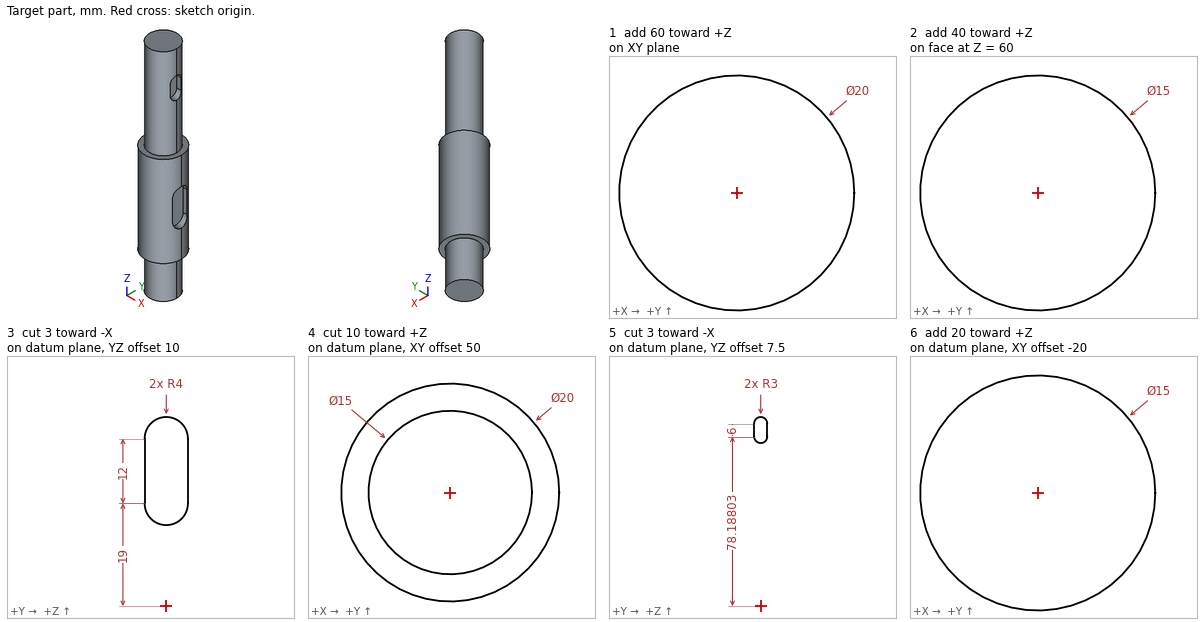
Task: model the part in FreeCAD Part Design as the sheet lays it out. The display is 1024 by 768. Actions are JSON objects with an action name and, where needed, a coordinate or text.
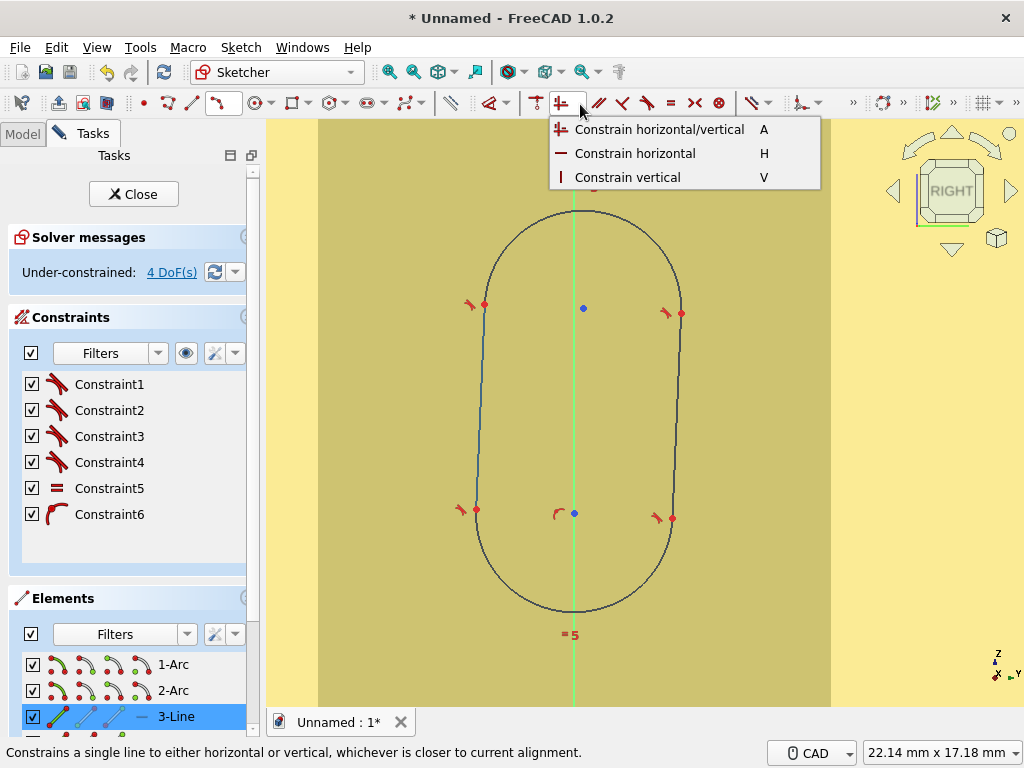
{"action": "left_click", "coordinate": [685, 177]}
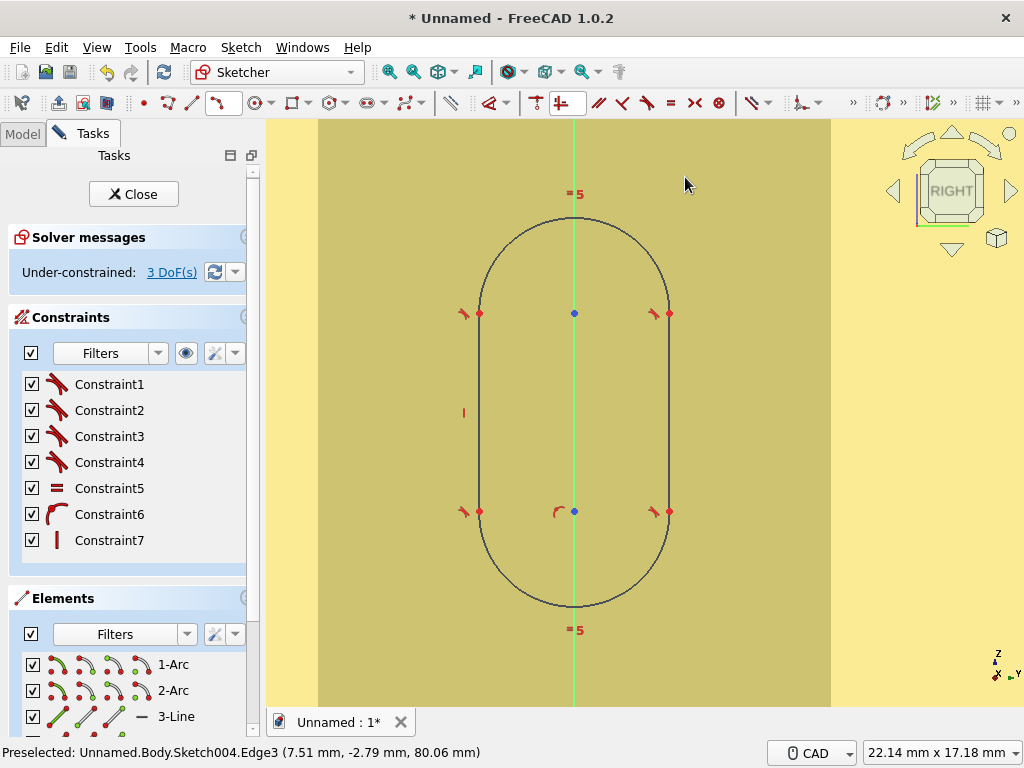
{"action": "left_click", "coordinate": [490, 104]}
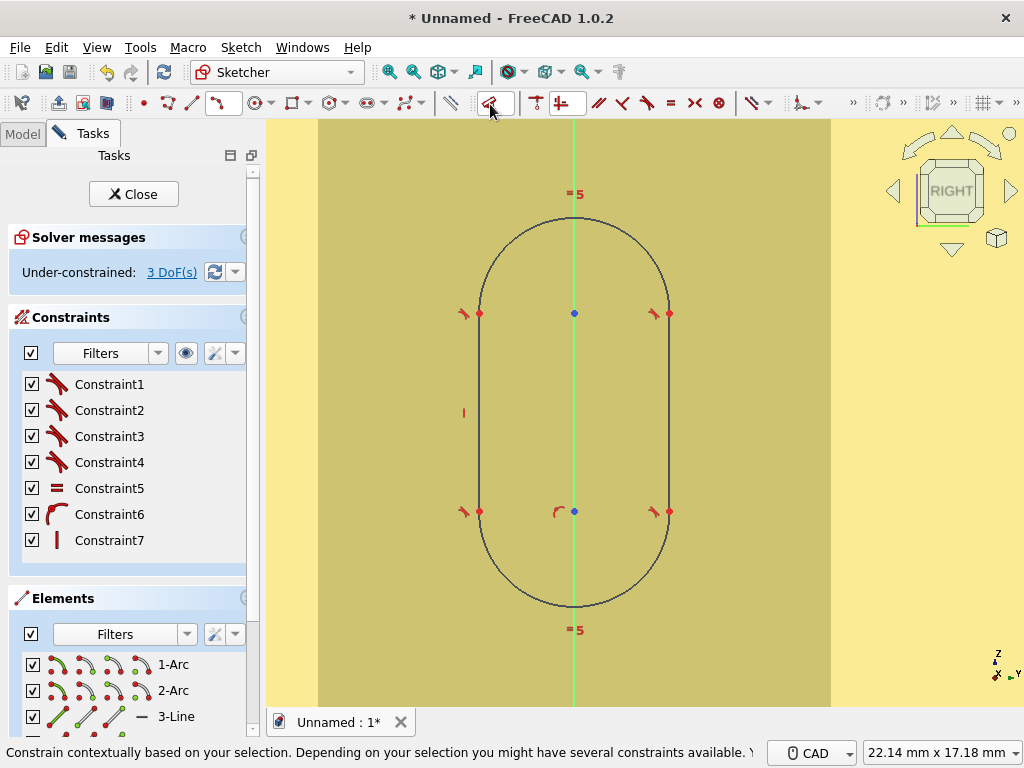
{"action": "left_click", "coordinate": [518, 589]}
{"action": "left_click", "coordinate": [499, 615]}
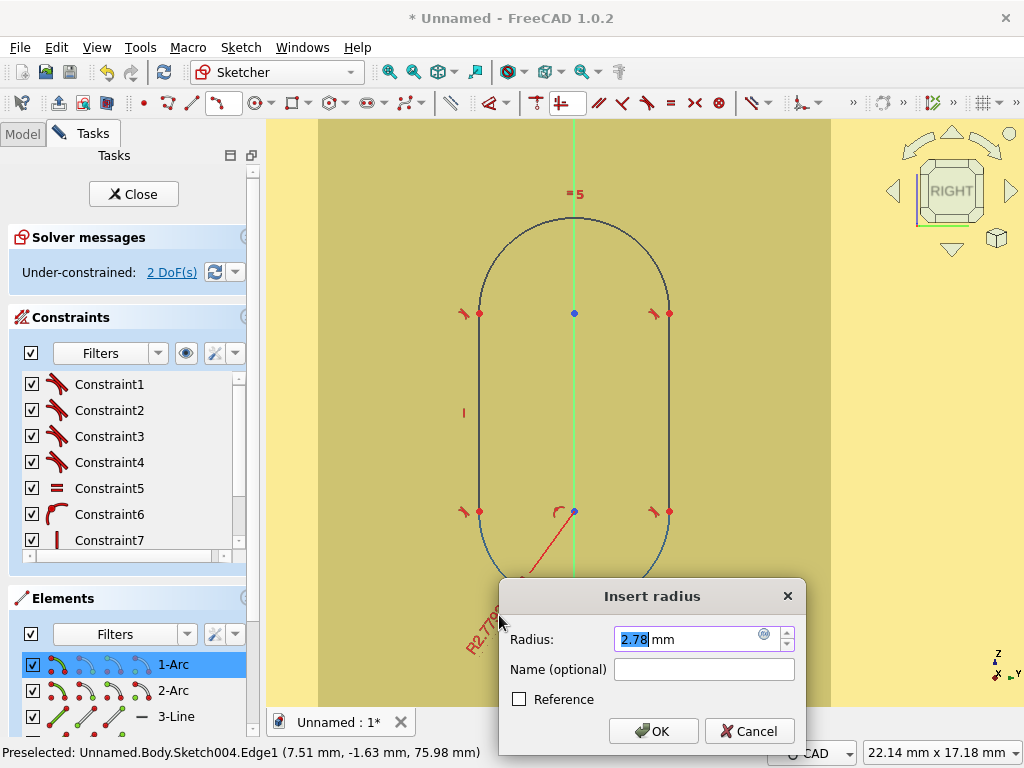
{"action": "type", "text": "3"}
{"action": "key", "text": "Return"}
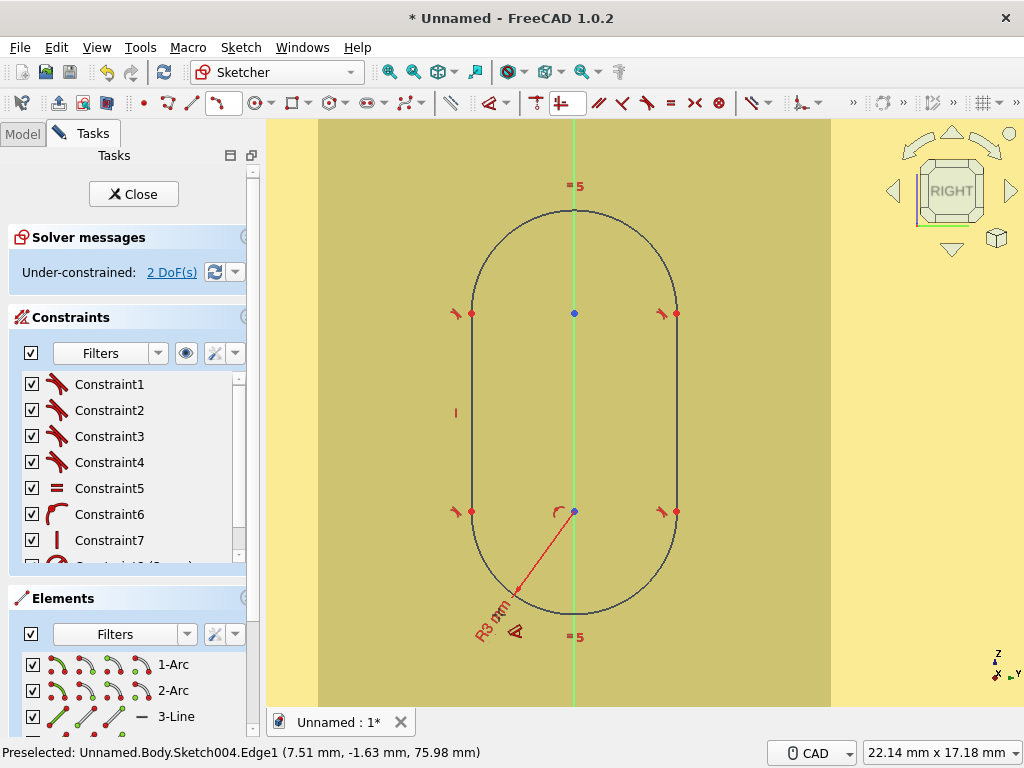
{"action": "left_click", "coordinate": [472, 452]}
{"action": "left_click", "coordinate": [438, 412]}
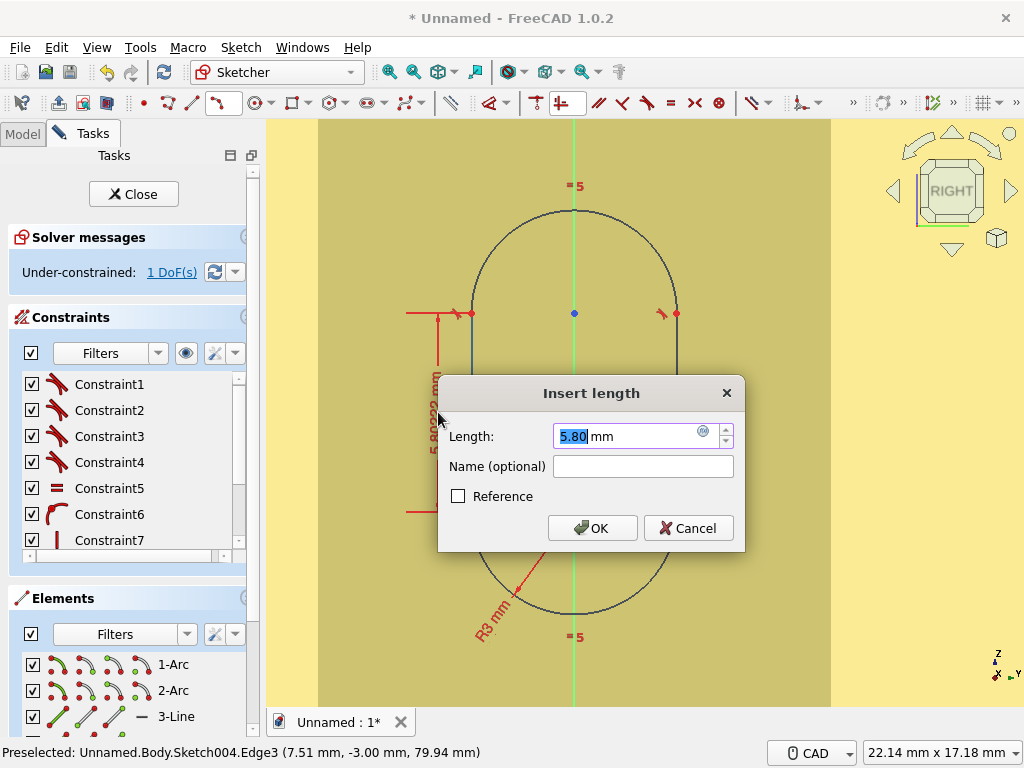
{"action": "type", "text": "6"}
{"action": "key", "text": "Return"}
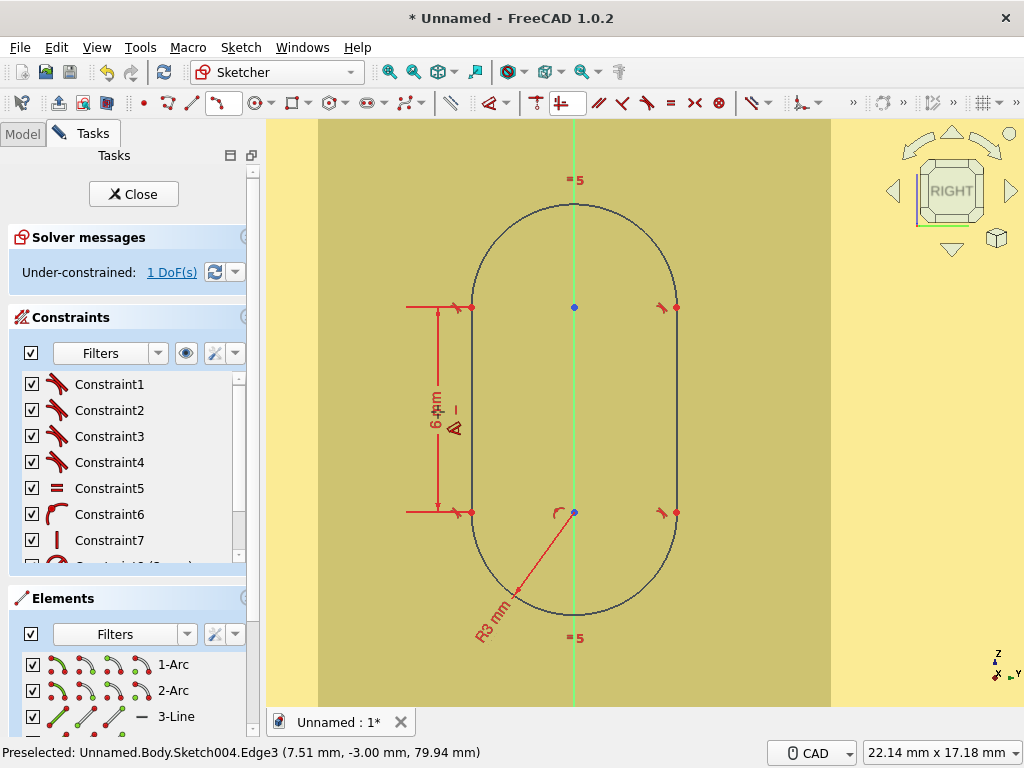
{"action": "left_click", "coordinate": [472, 512]}
{"action": "left_click", "coordinate": [438, 557]}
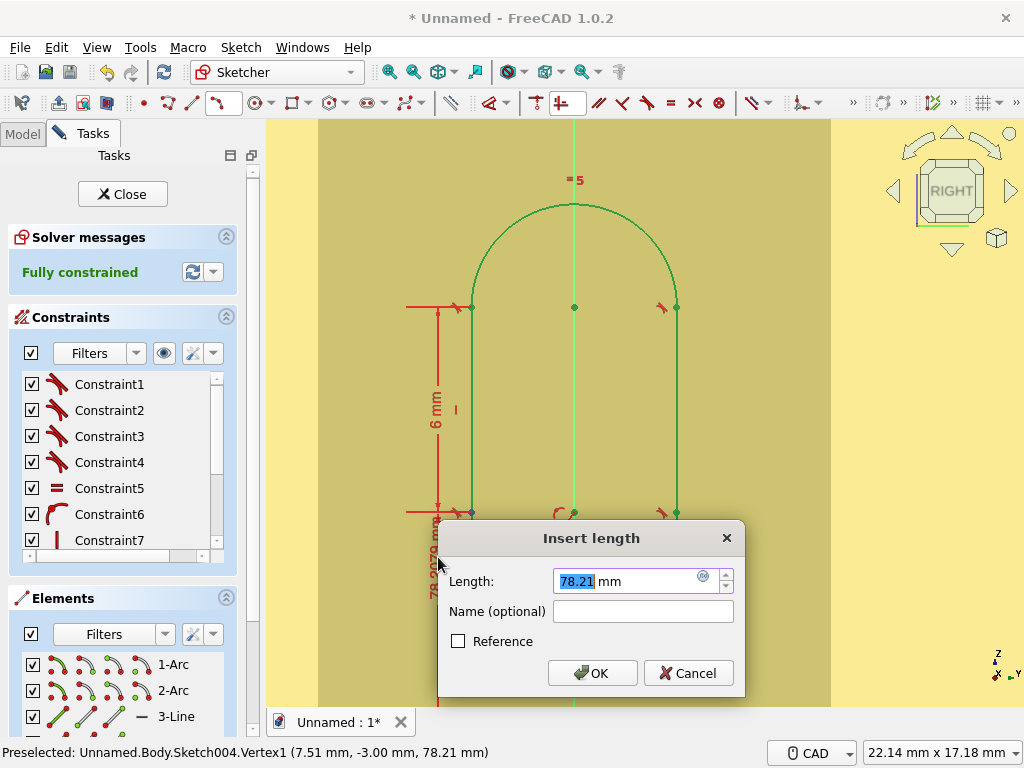
{"action": "type", "text": "78.18803"}
{"action": "key", "text": "Return"}
{"action": "key", "text": "Escape"}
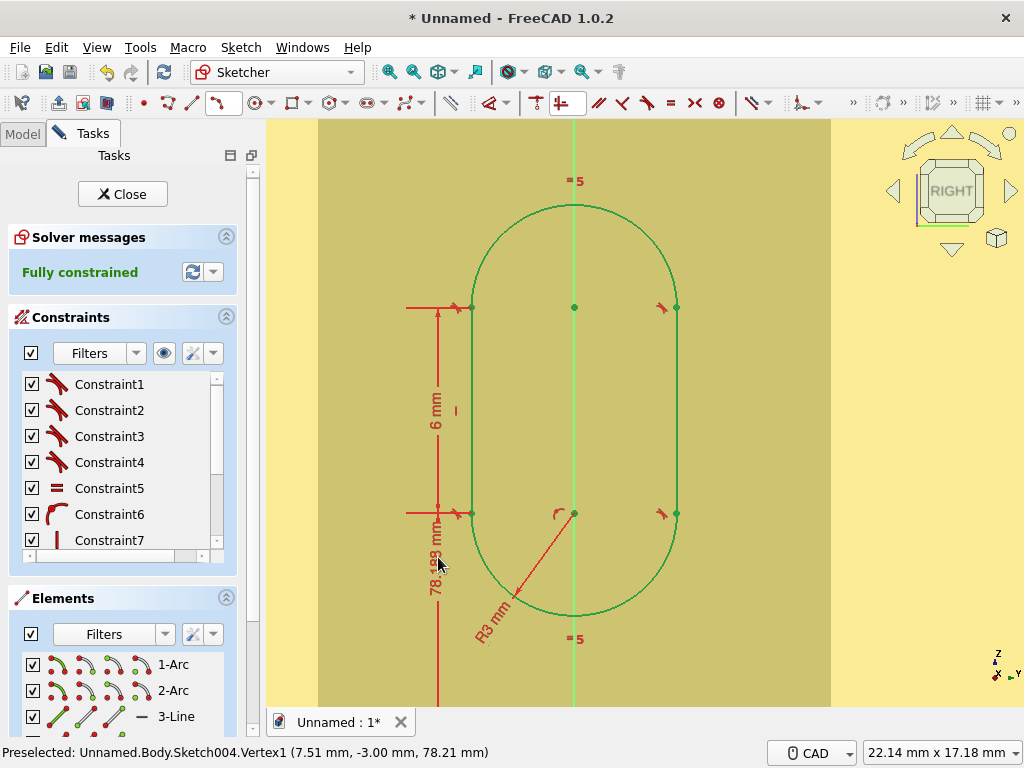
{"action": "left_click", "coordinate": [123, 194]}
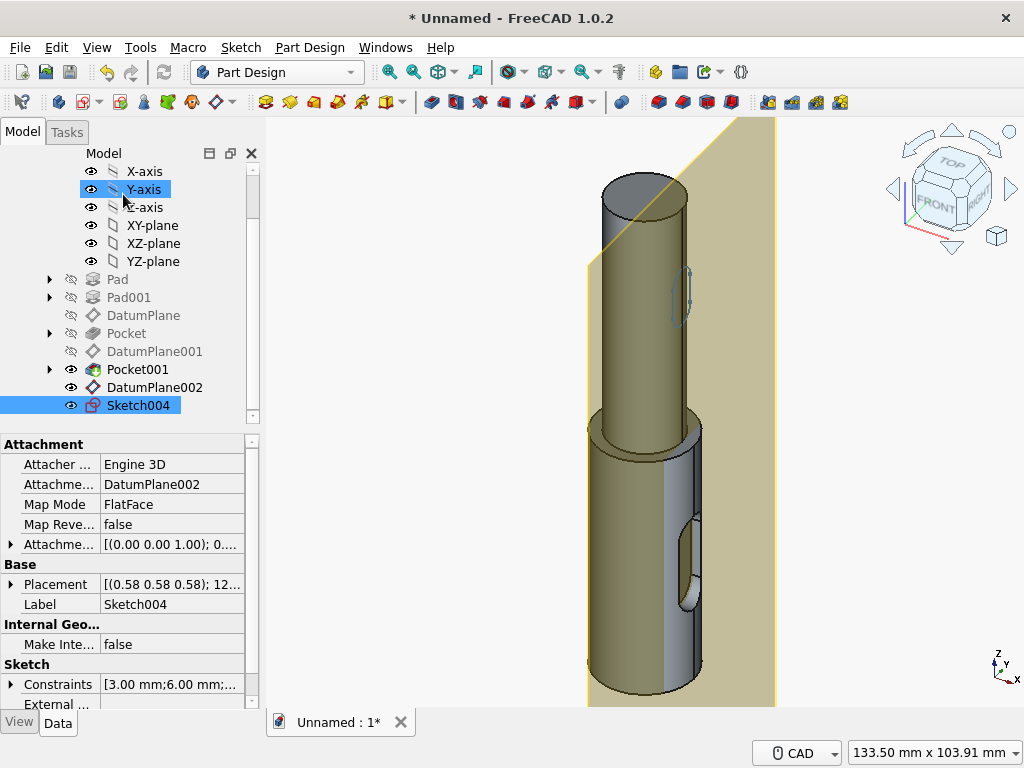
{"action": "left_click", "coordinate": [432, 102]}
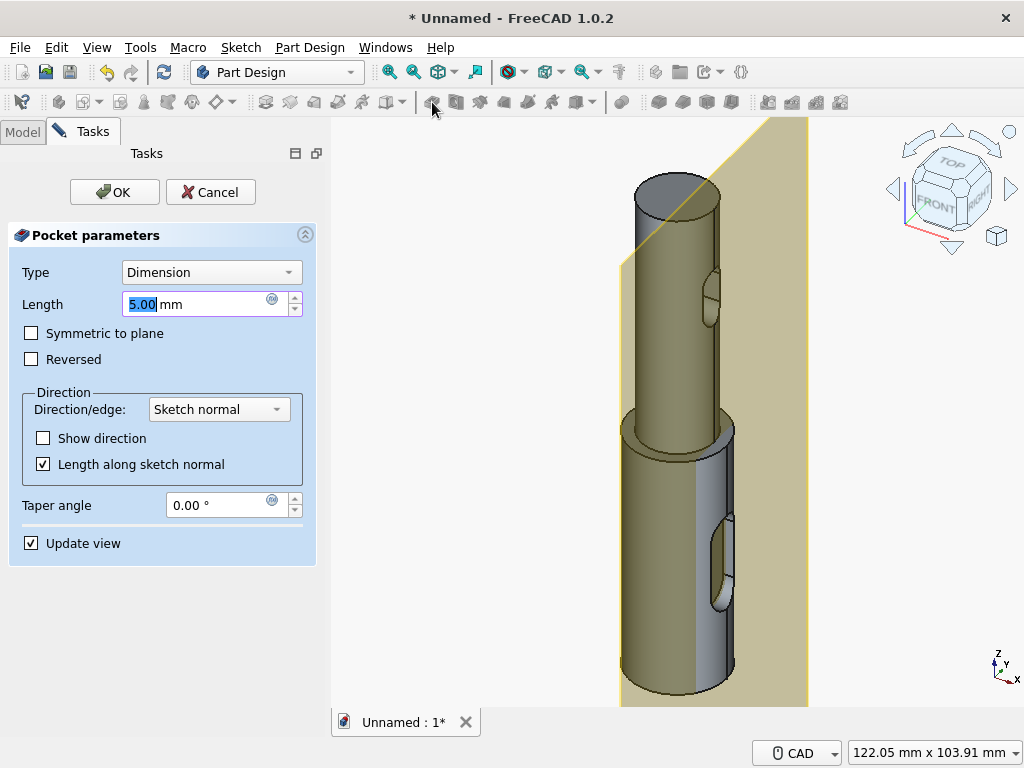
{"action": "type", "text": "3"}
{"action": "key", "text": "Tab"}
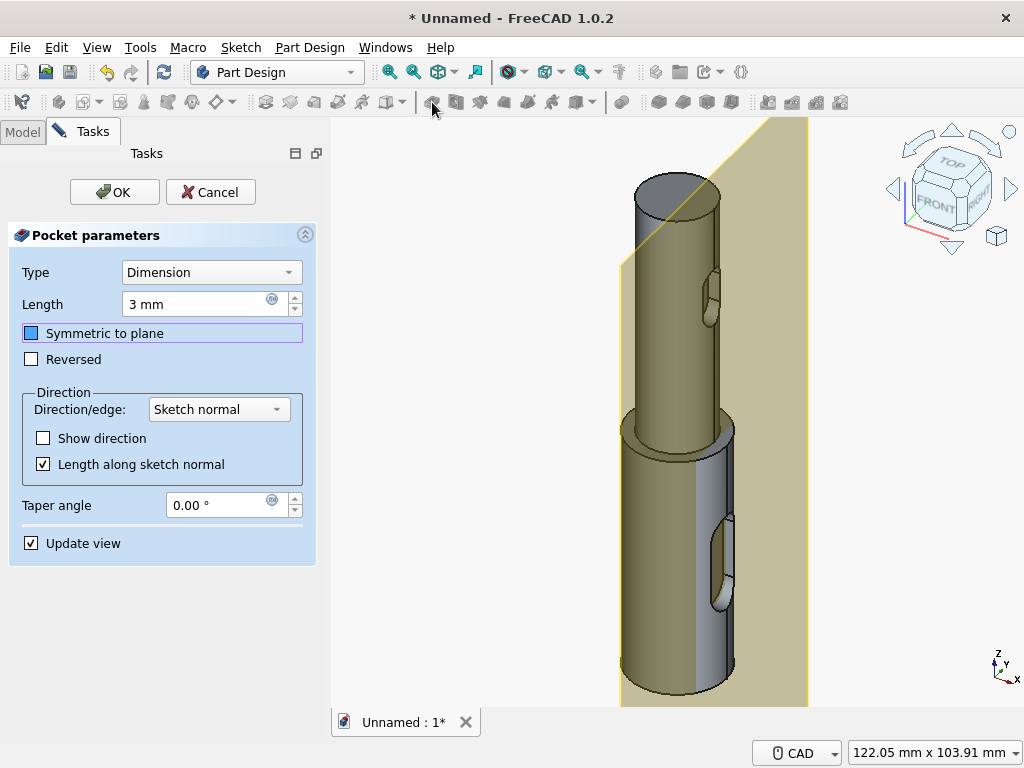
{"action": "left_click", "coordinate": [115, 192]}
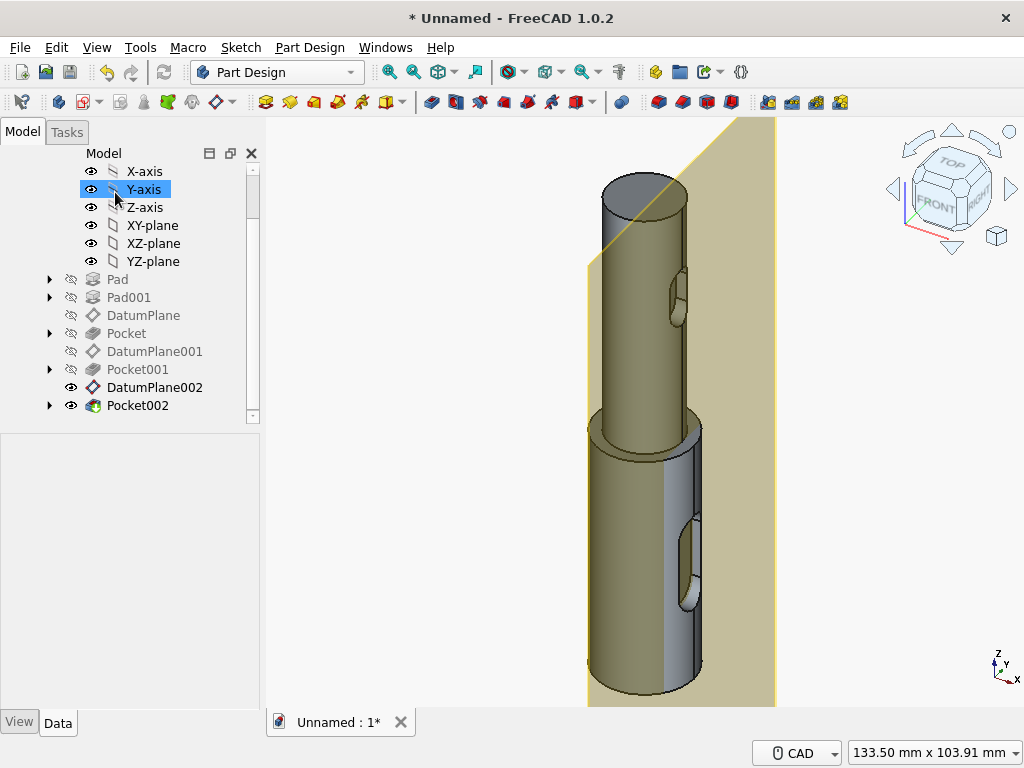
{"action": "left_click", "coordinate": [116, 387]}
{"action": "key", "text": "space"}